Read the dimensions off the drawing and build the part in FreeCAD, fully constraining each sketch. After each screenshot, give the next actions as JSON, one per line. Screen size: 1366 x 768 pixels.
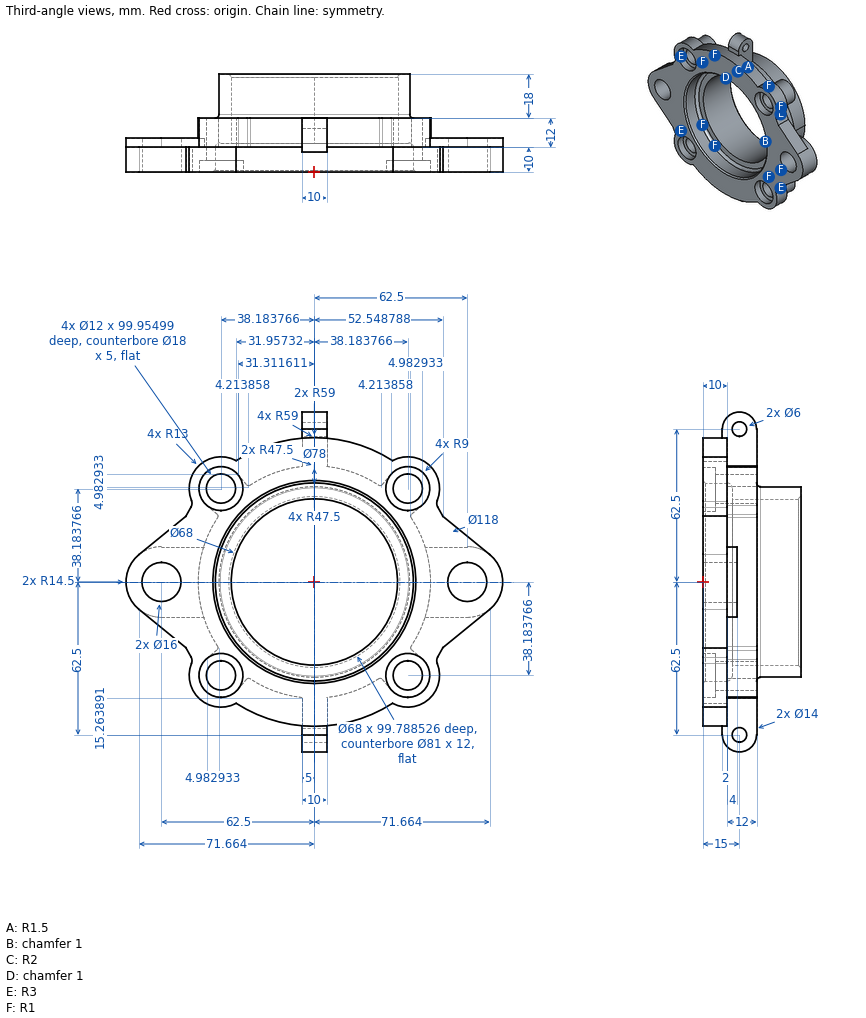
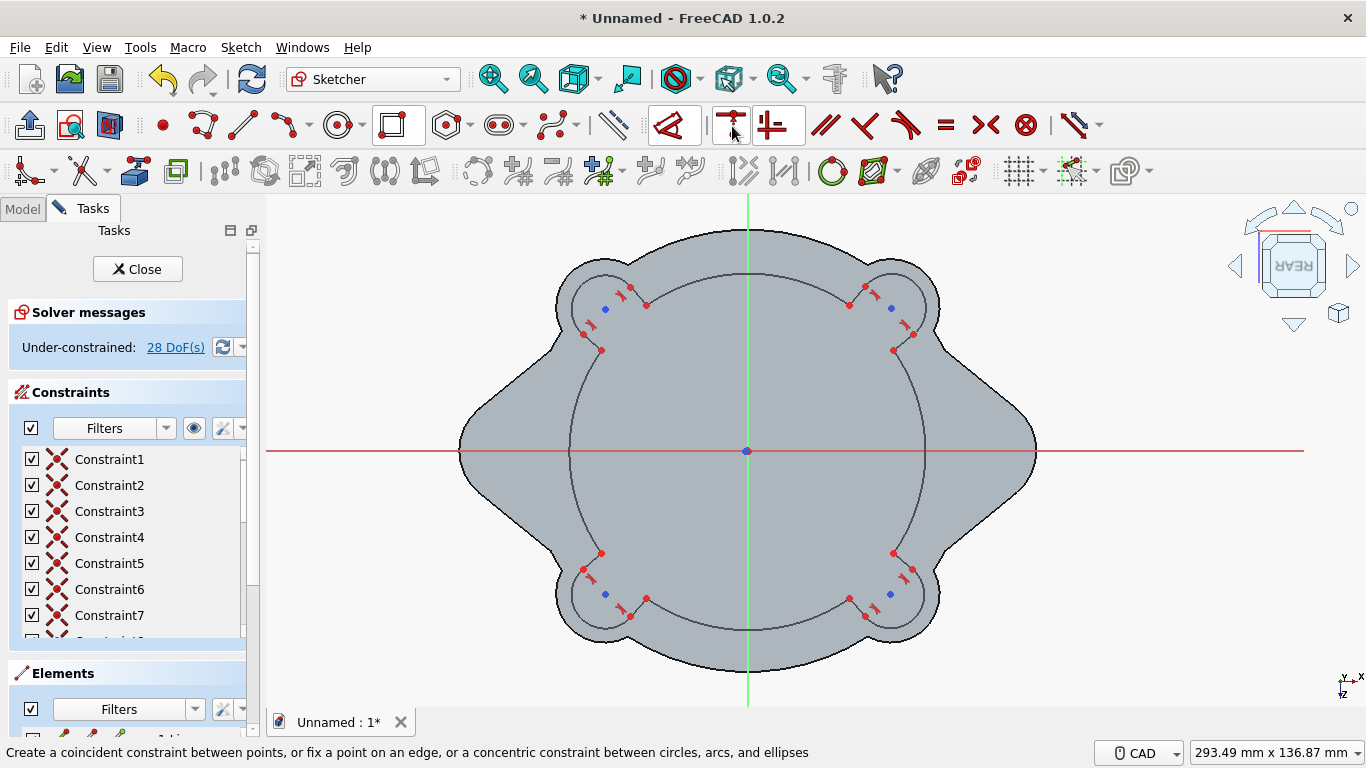
{"action": "left_click", "coordinate": [705, 625]}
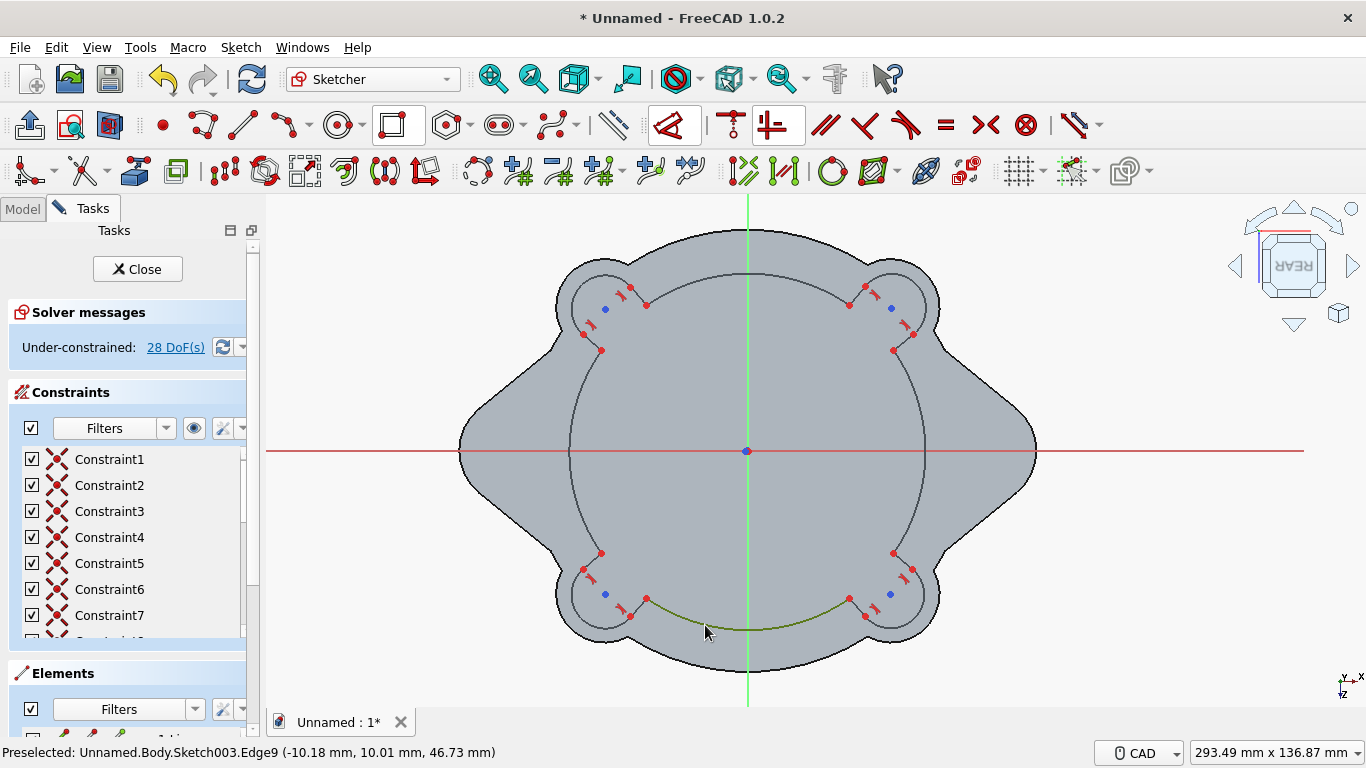
{"action": "left_click", "coordinate": [575, 409]}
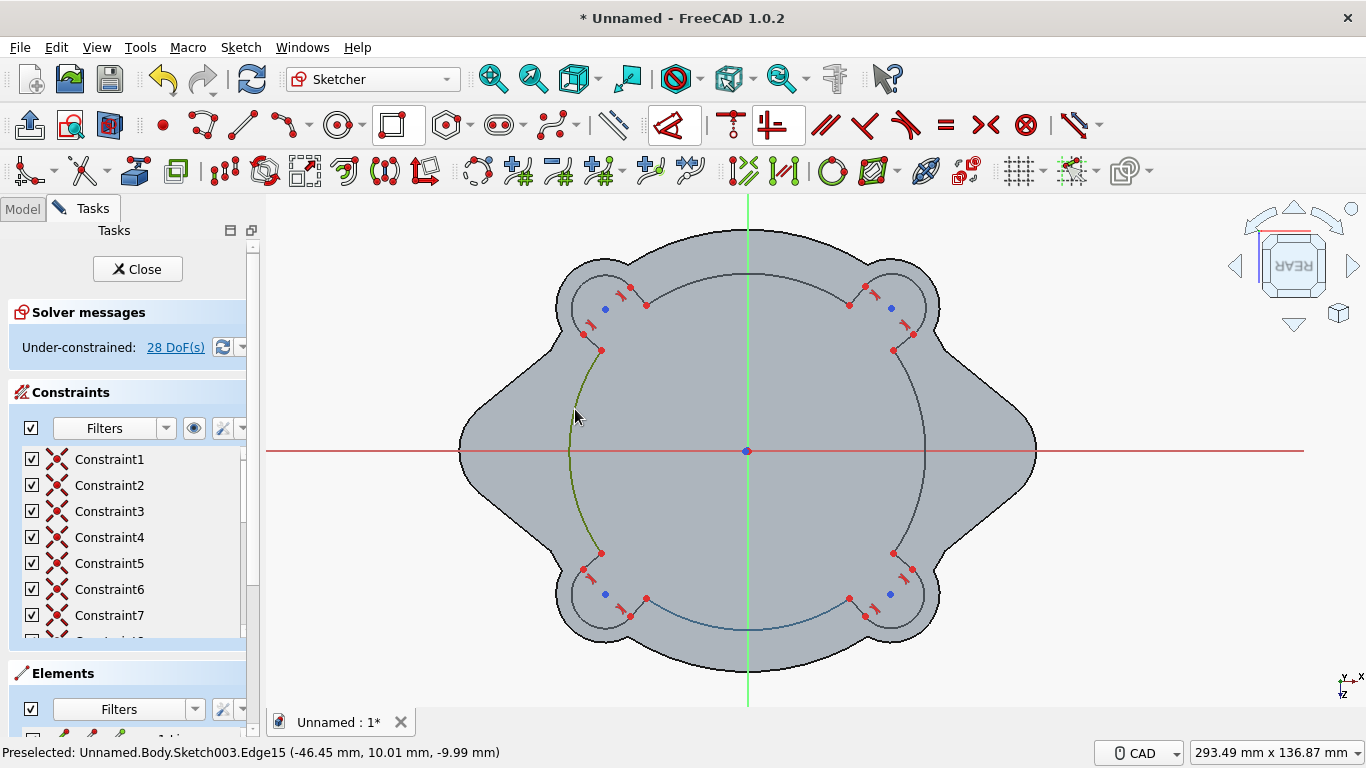
{"action": "left_click", "coordinate": [732, 126]}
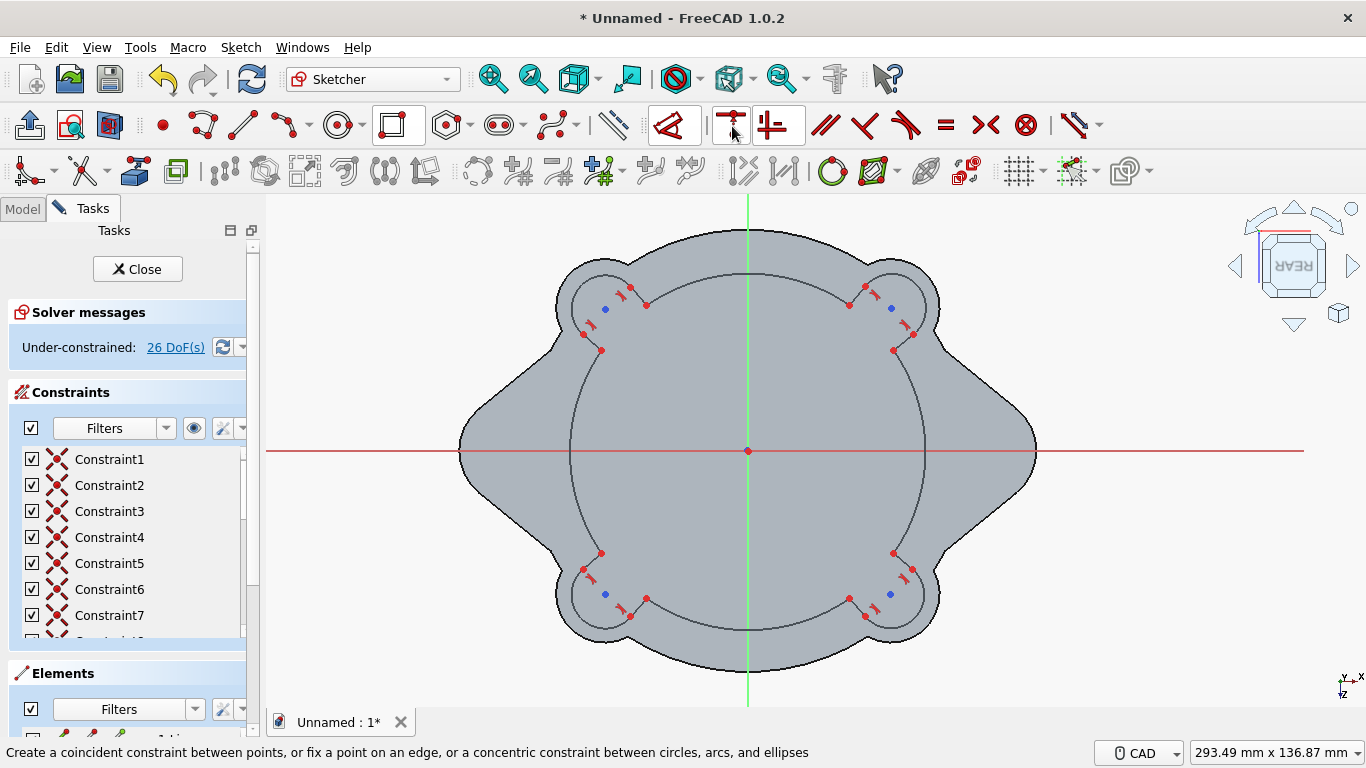
{"action": "left_click_drag", "start_coordinate": [738, 441], "coordinate": [758, 462]}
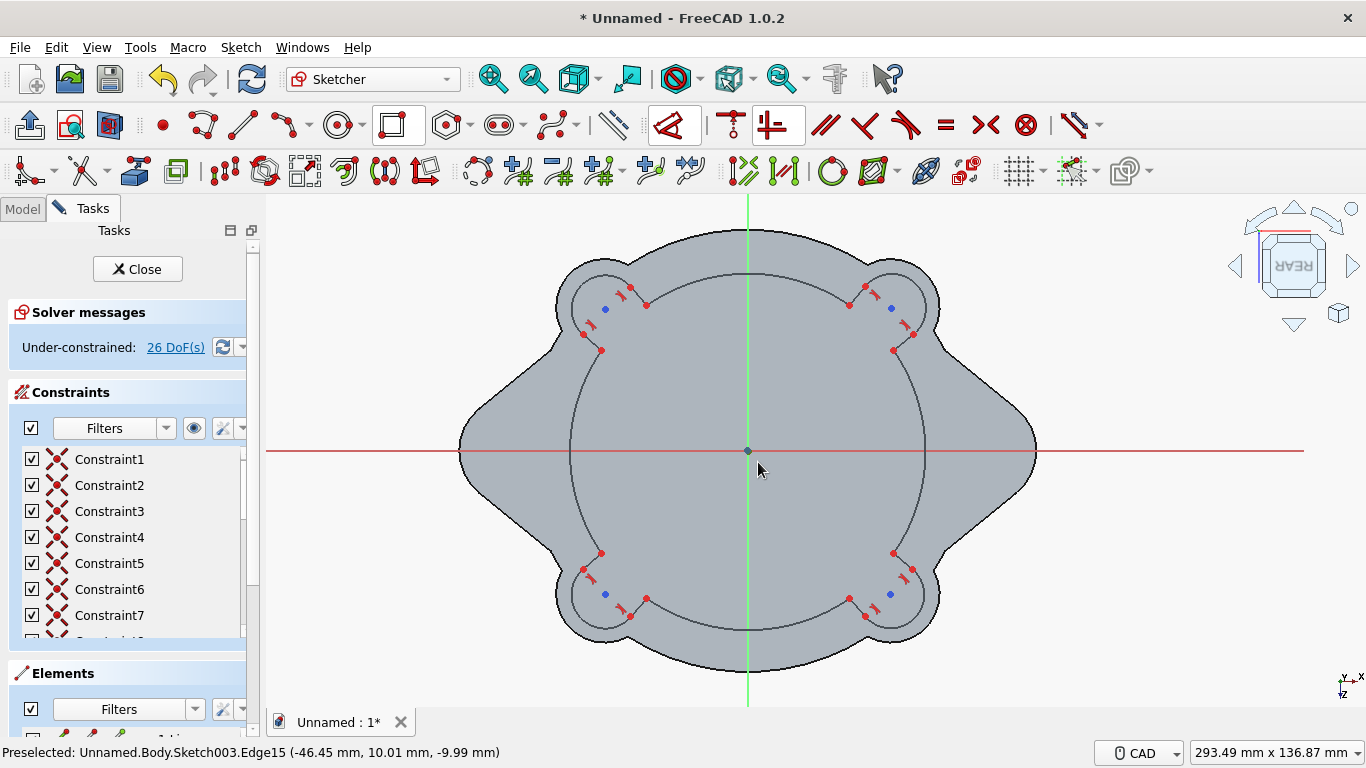
{"action": "left_click", "coordinate": [732, 126]}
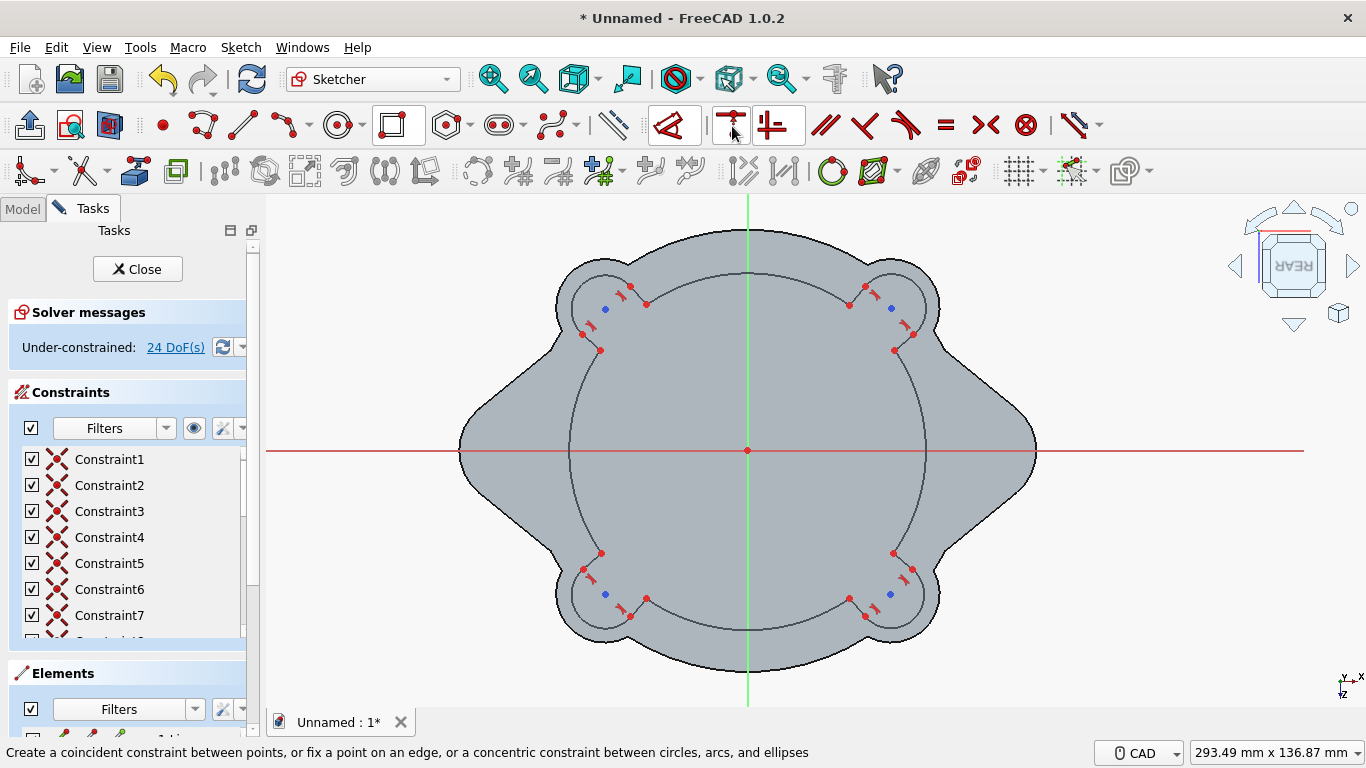
{"action": "left_click", "coordinate": [705, 625]}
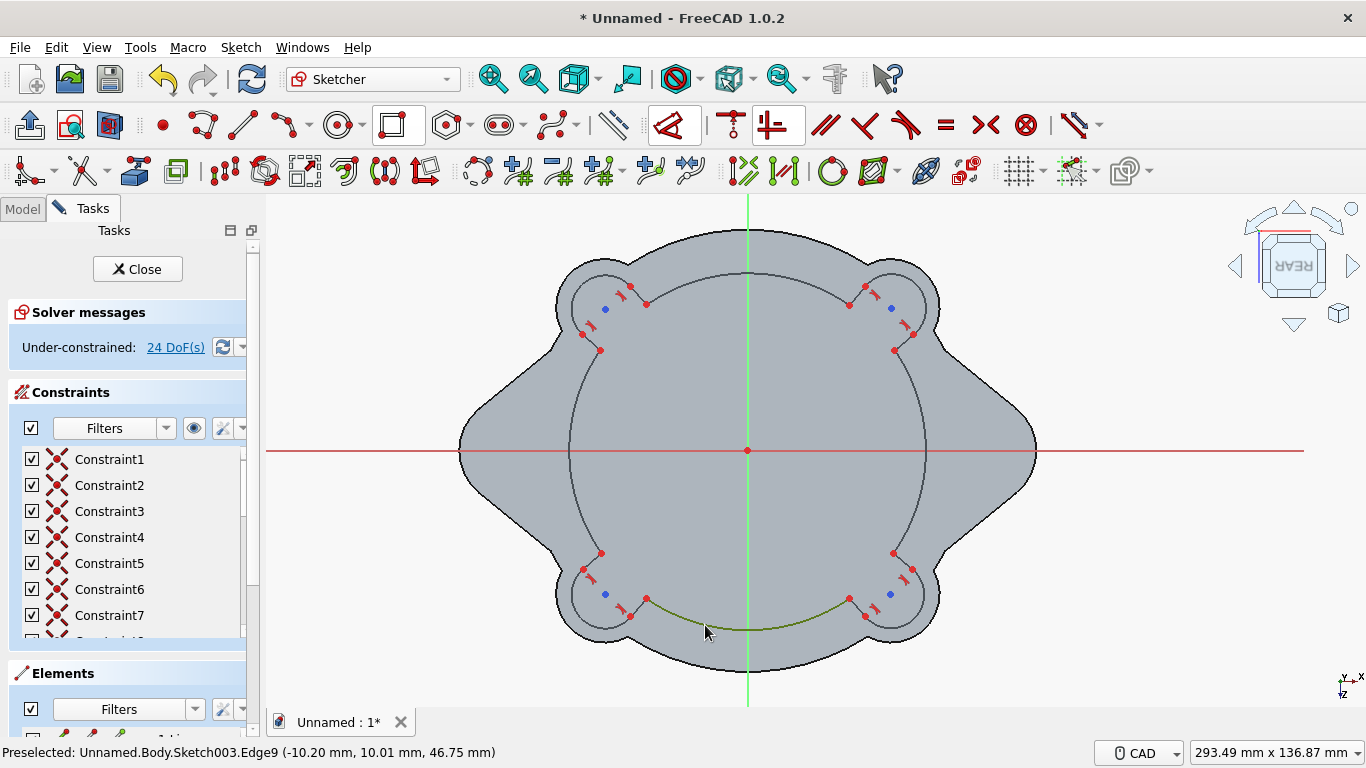
{"action": "left_click", "coordinate": [920, 495]}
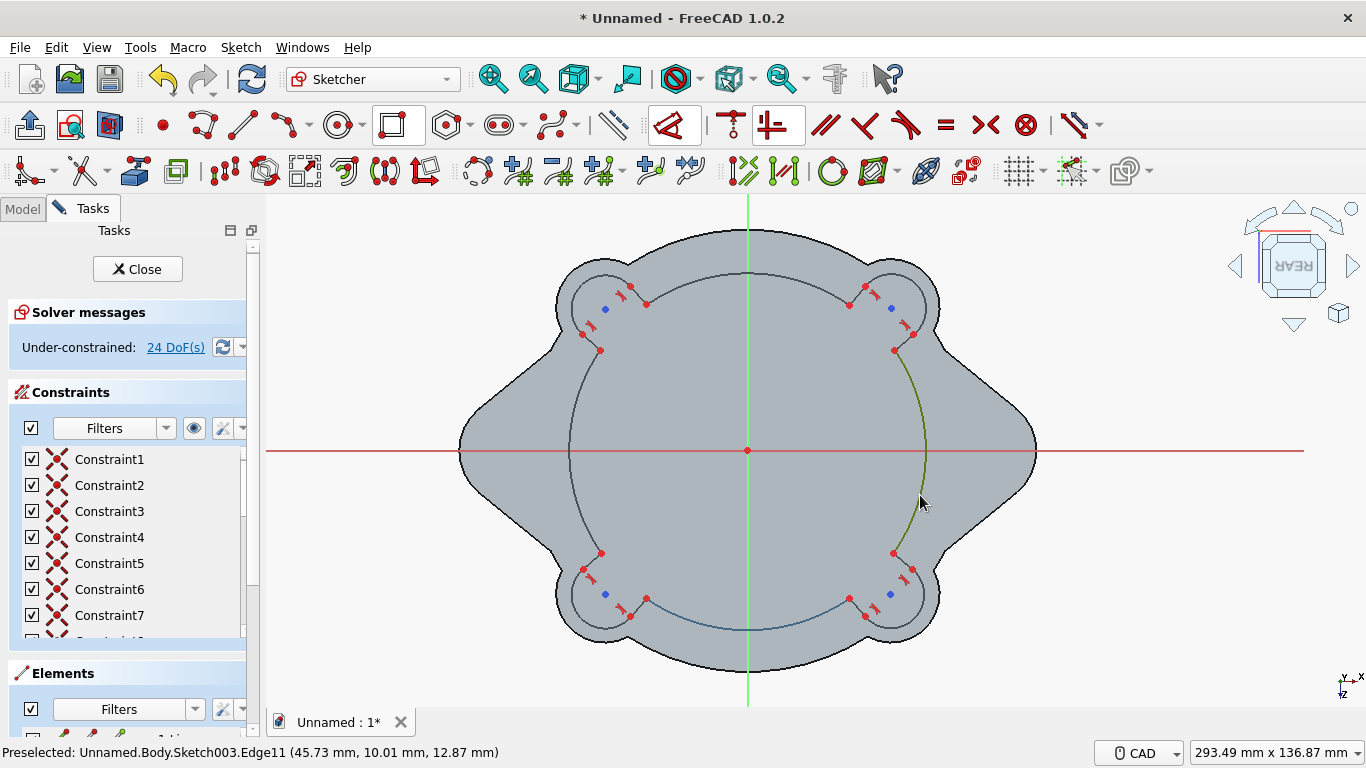
{"action": "left_click", "coordinate": [791, 279]}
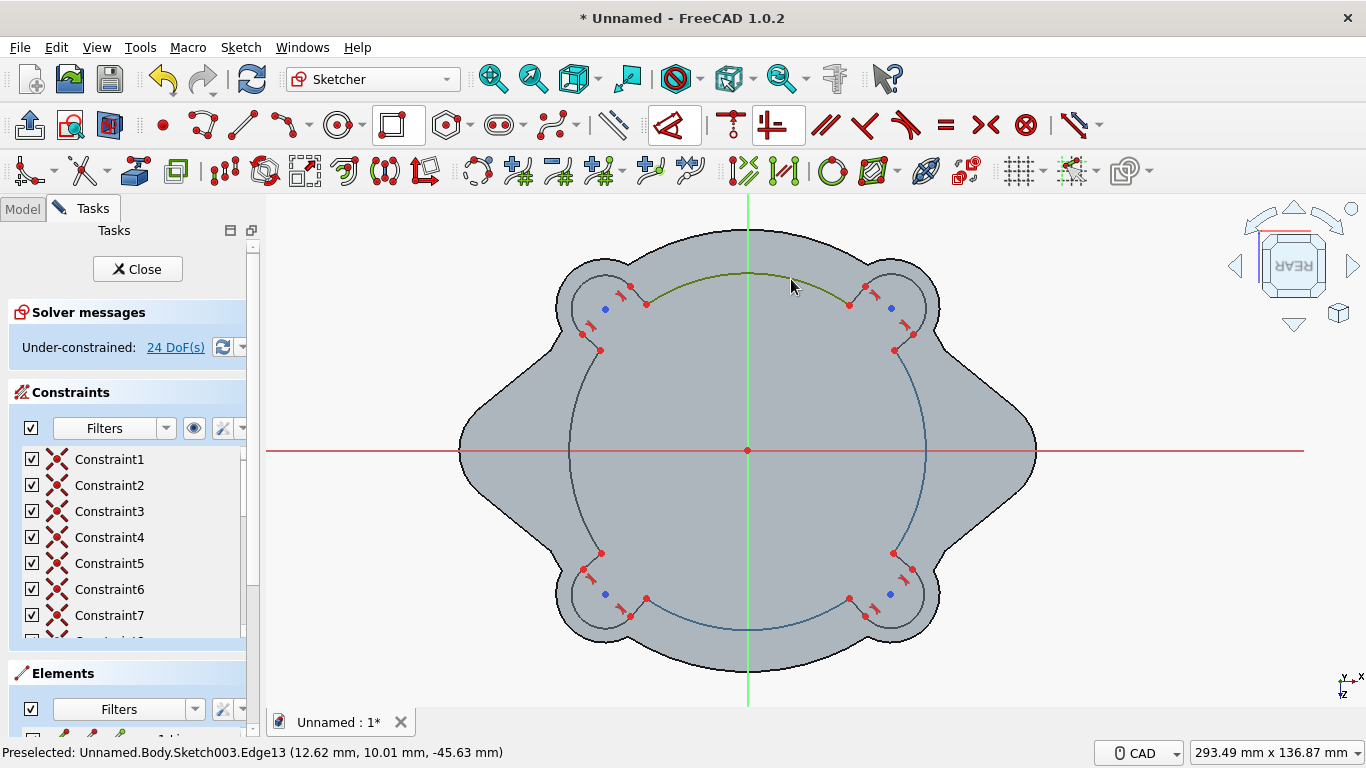
{"action": "left_click", "coordinate": [574, 409]}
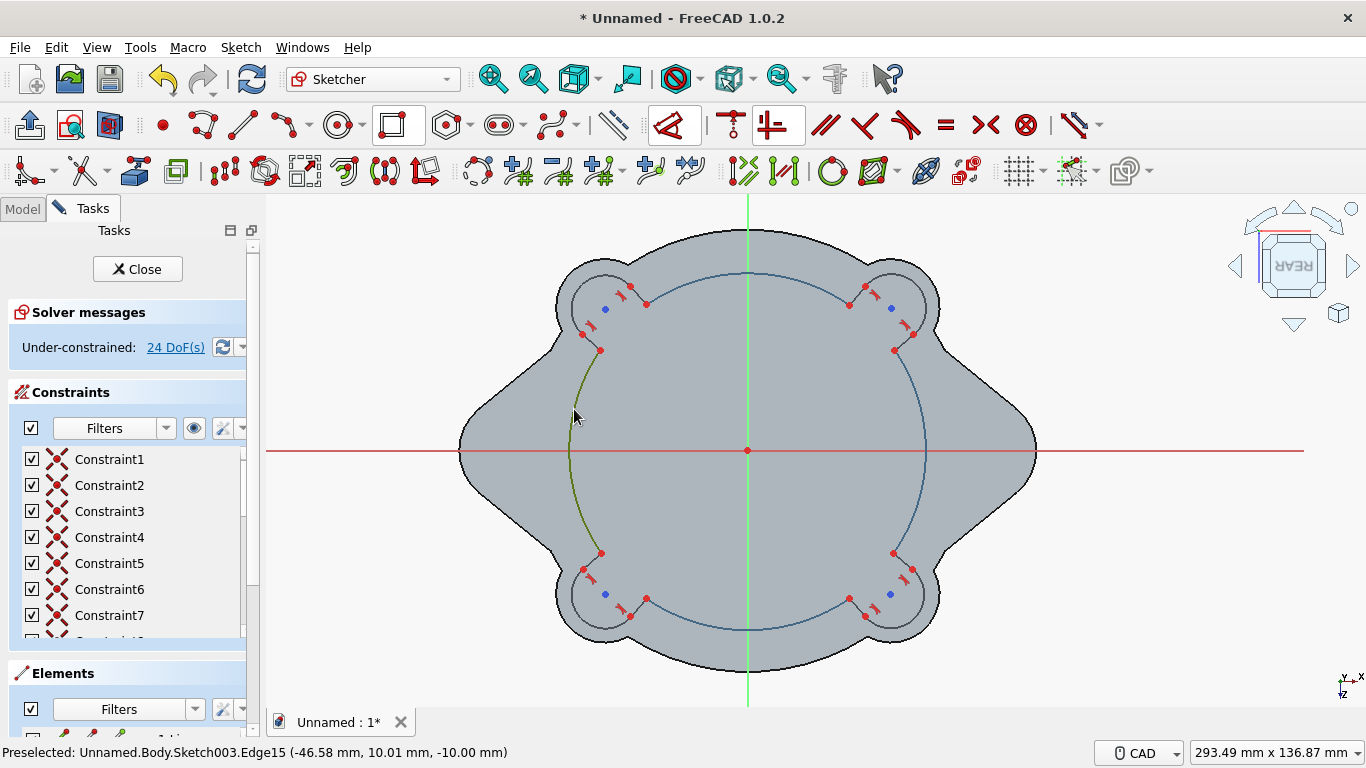
{"action": "left_click", "coordinate": [946, 126]}